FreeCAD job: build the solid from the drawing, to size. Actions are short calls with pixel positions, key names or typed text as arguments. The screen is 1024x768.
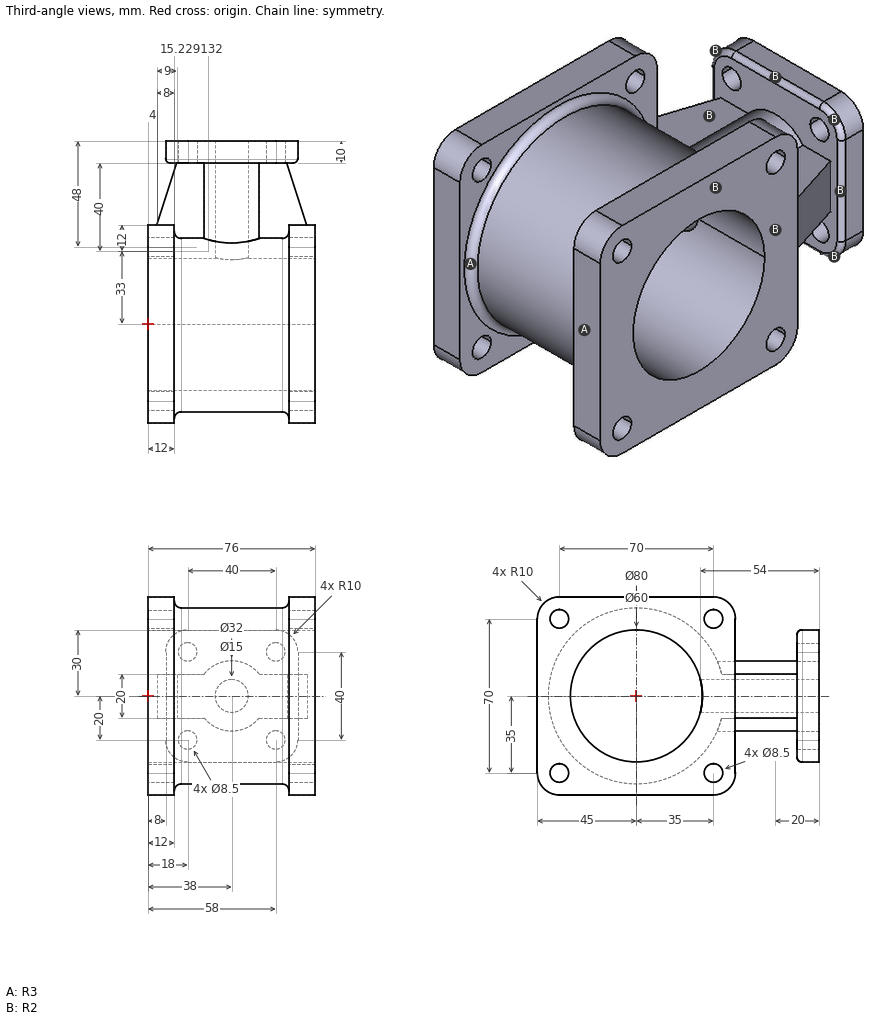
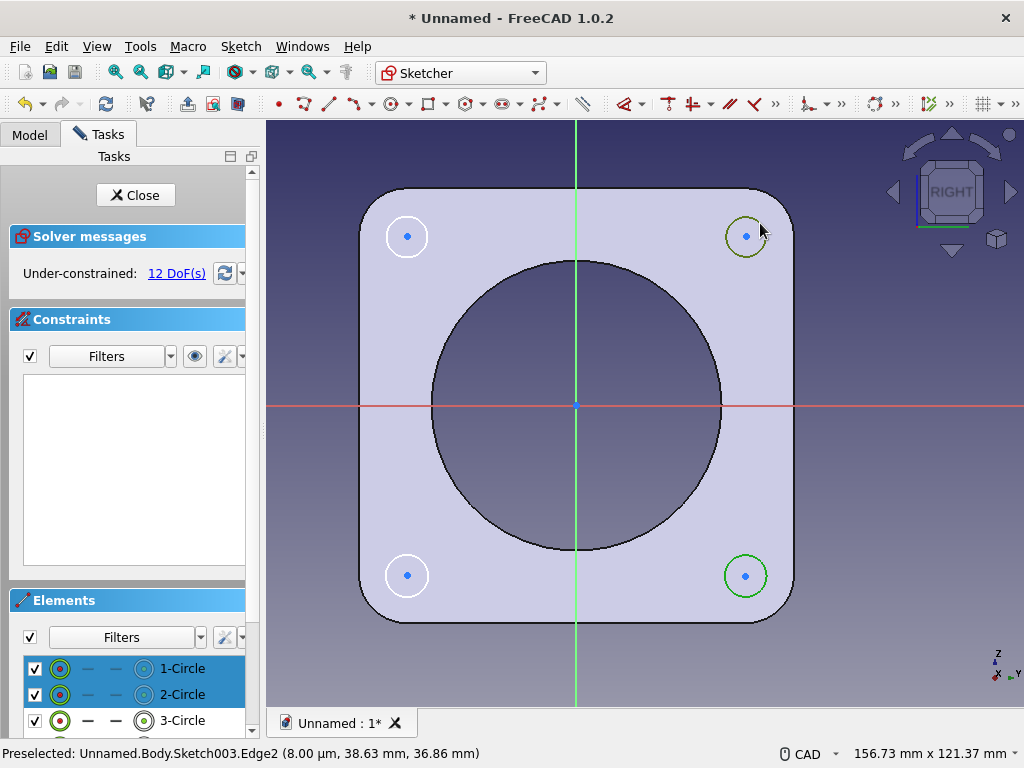
click(422, 561)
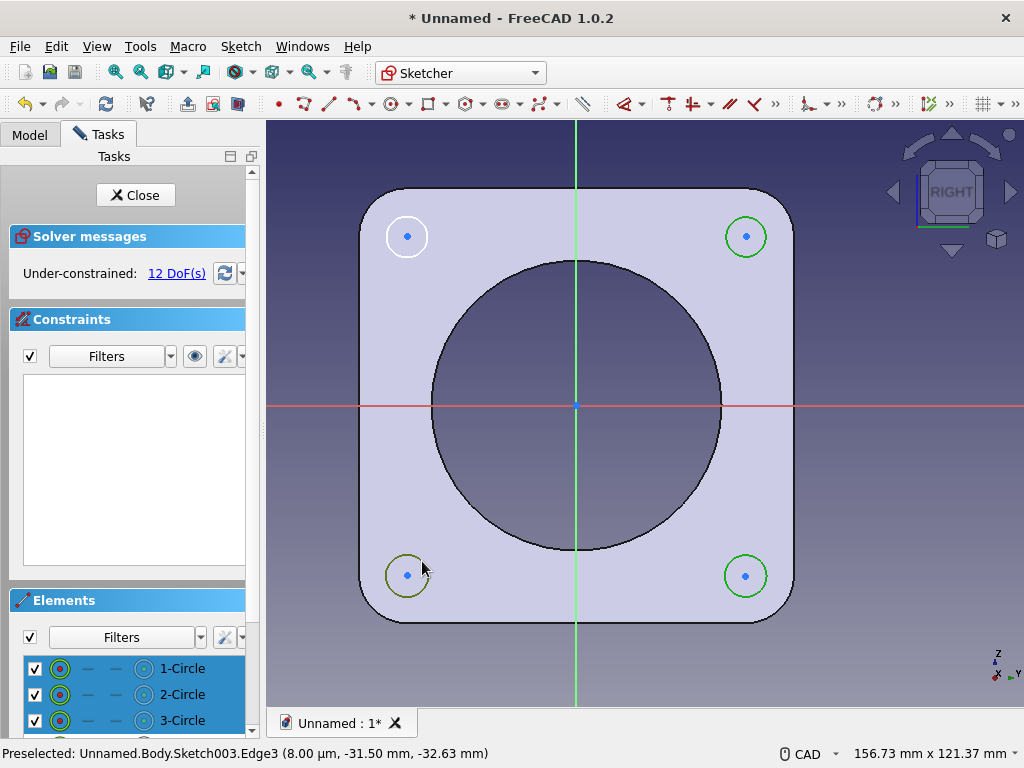
click(421, 222)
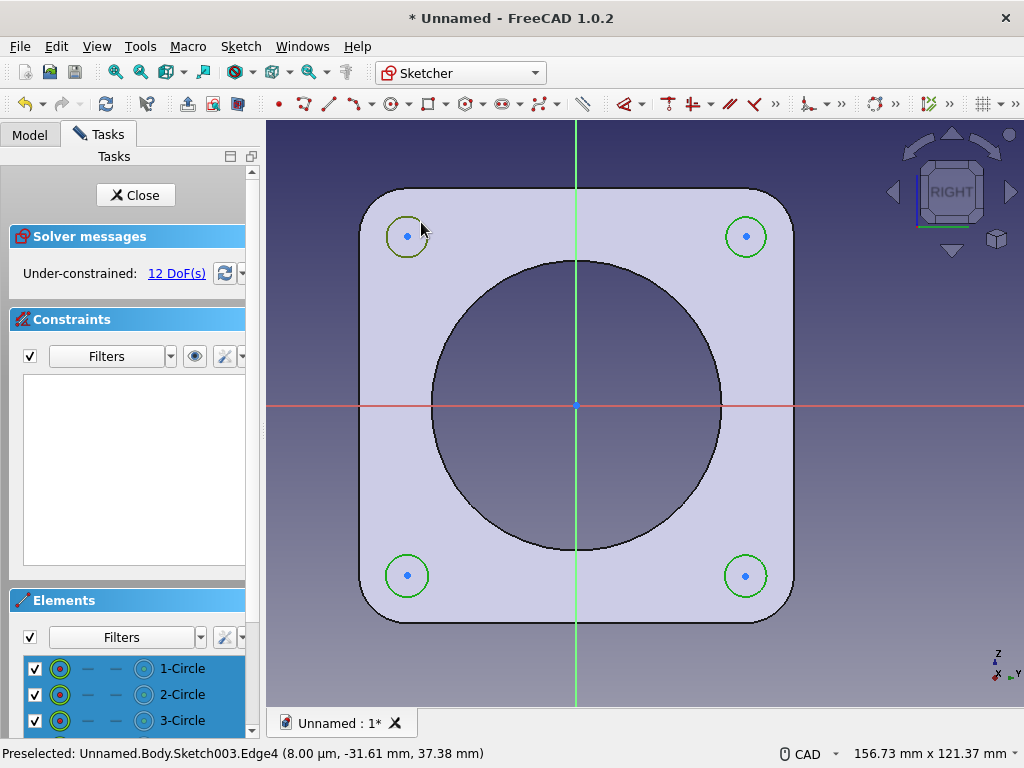
key(e)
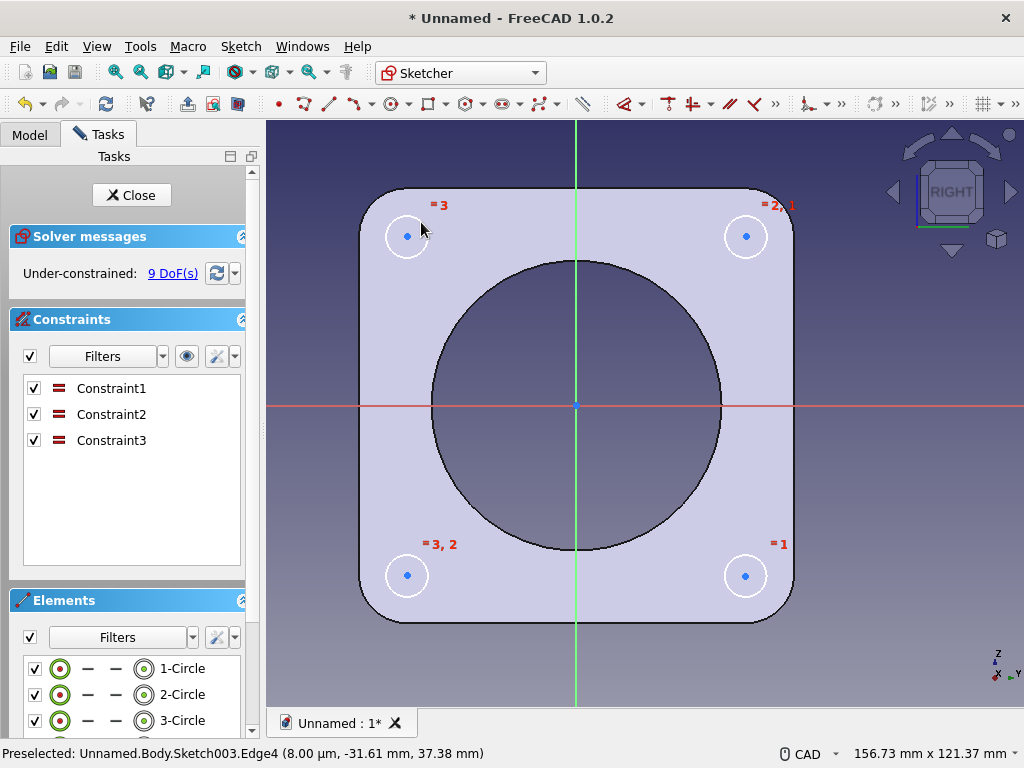
click(746, 576)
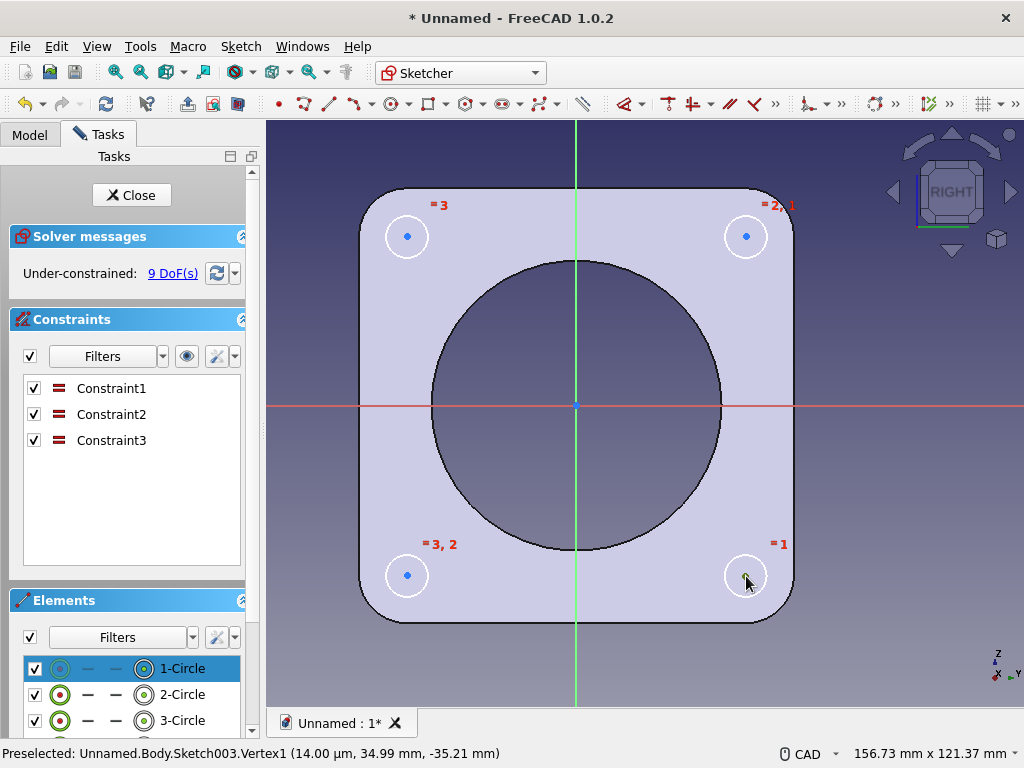
click(746, 237)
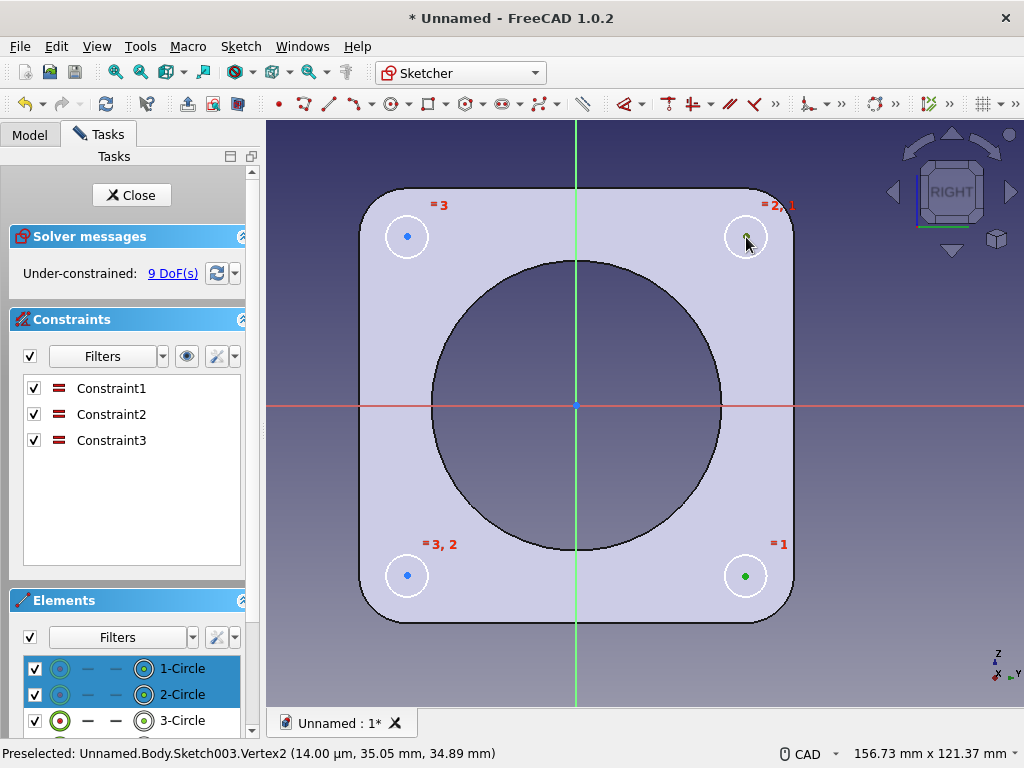
click(334, 406)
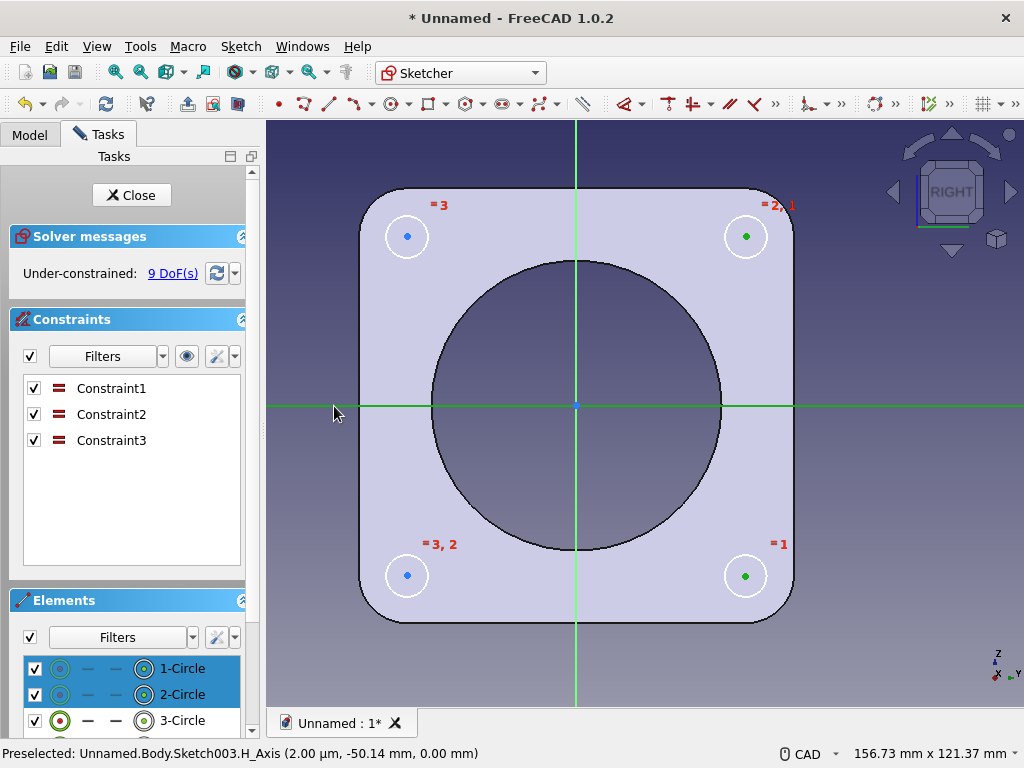
key(s)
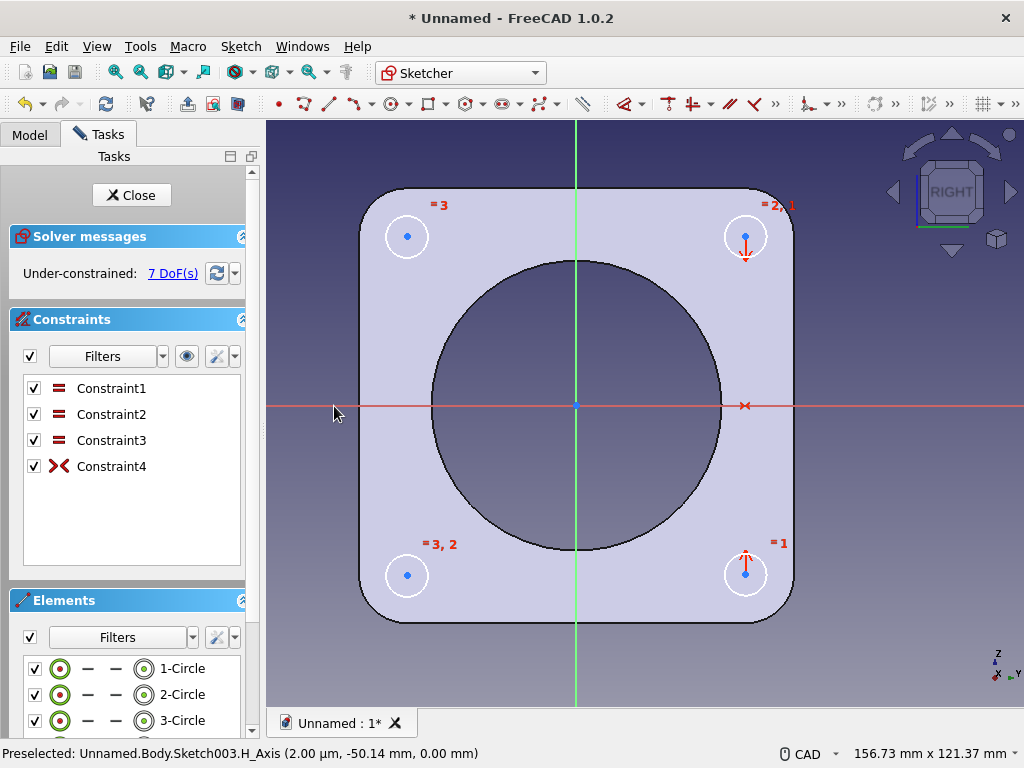
click(746, 575)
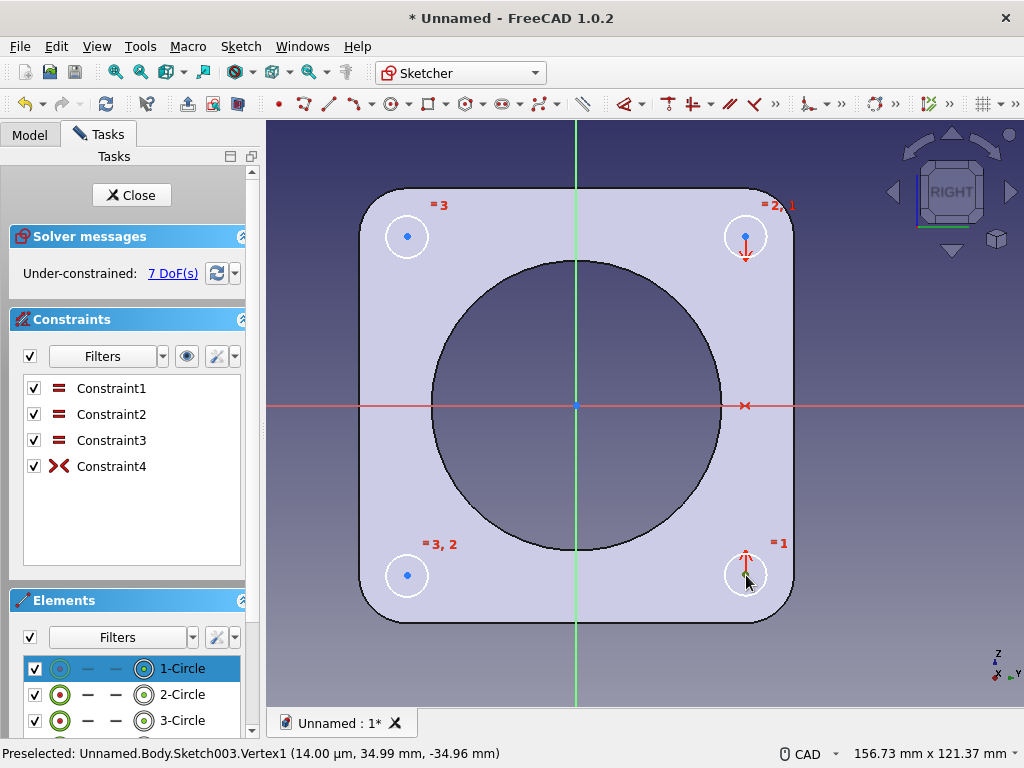
click(407, 576)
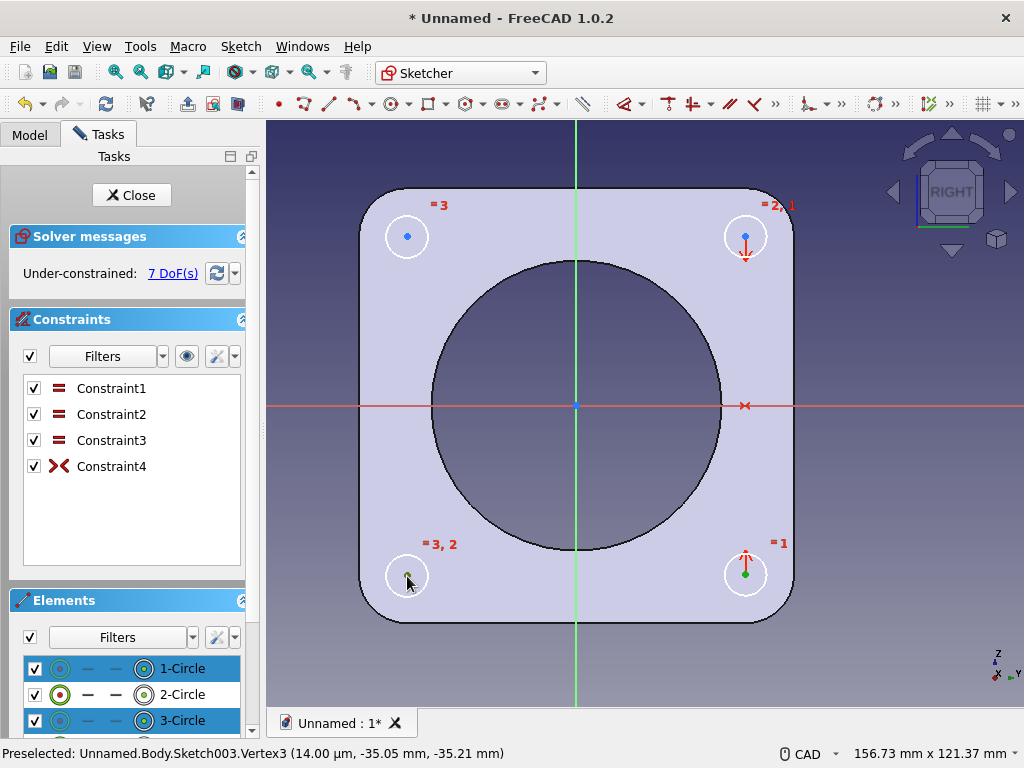
click(577, 641)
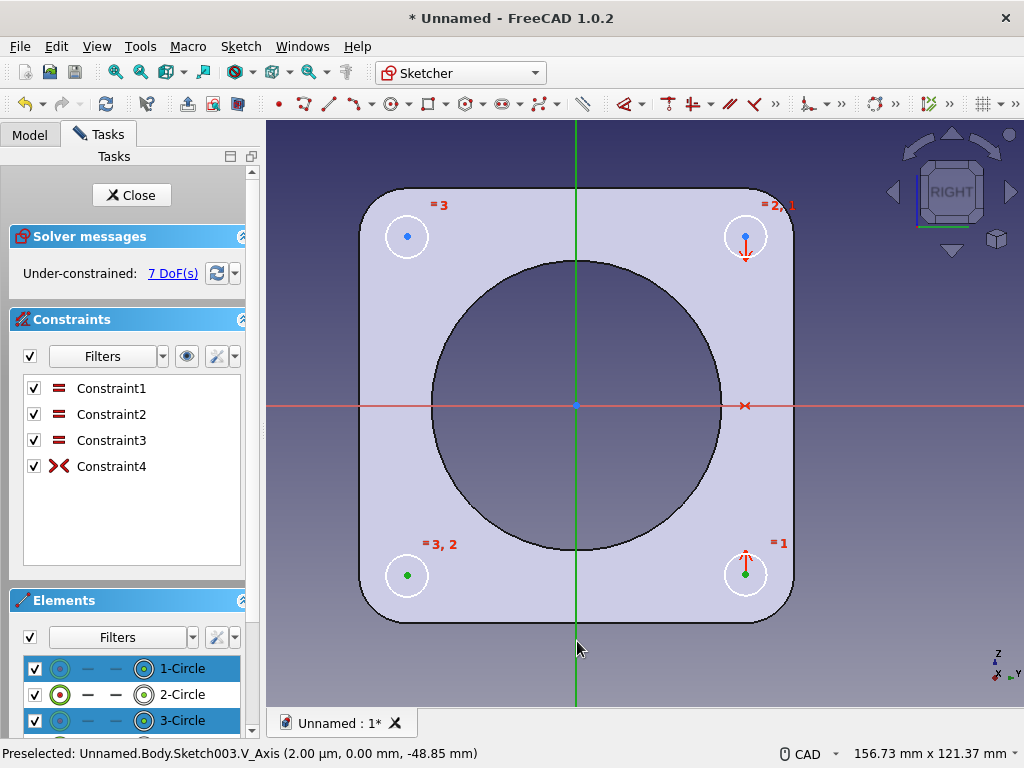
key(s)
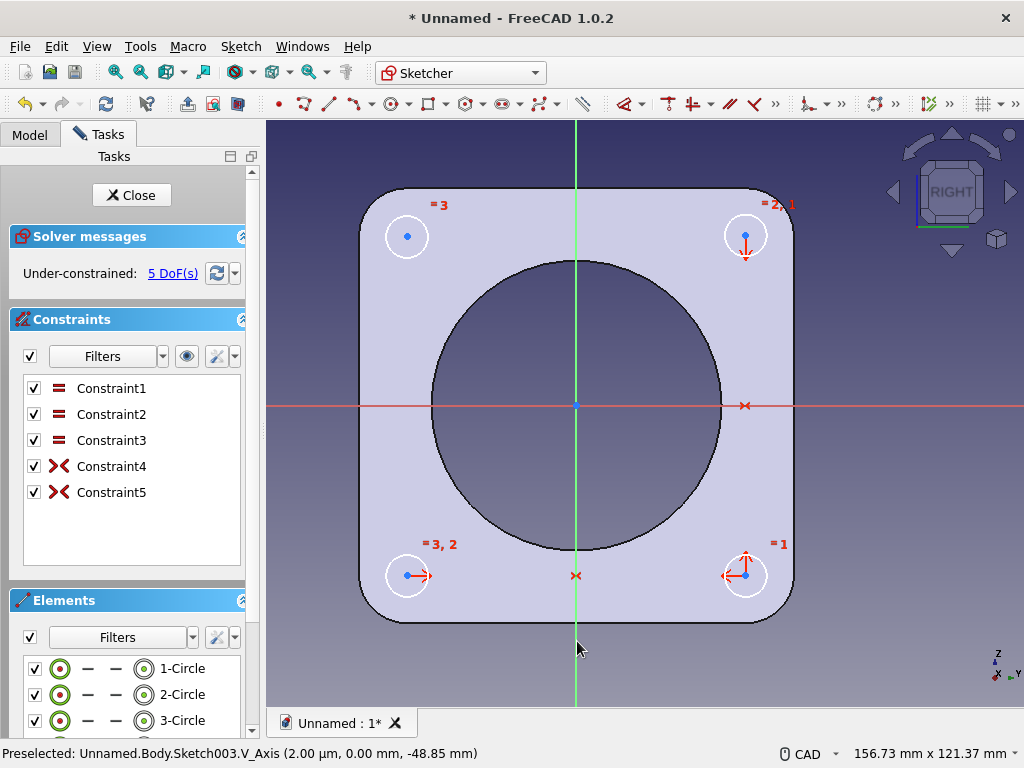
click(746, 235)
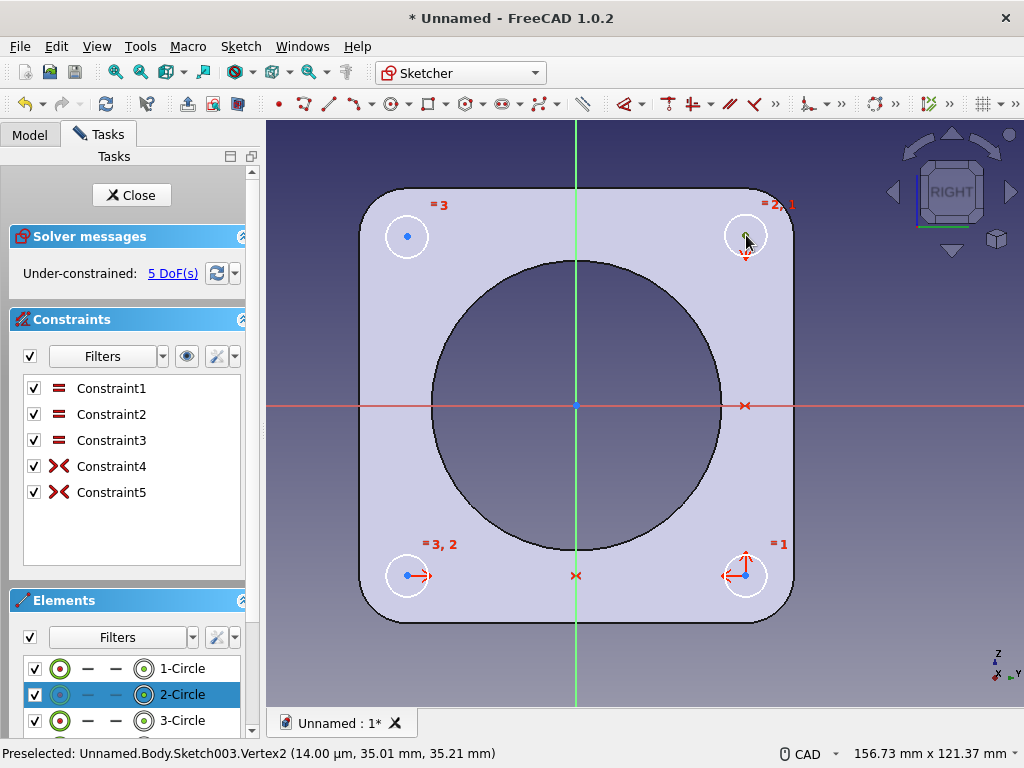
click(407, 237)